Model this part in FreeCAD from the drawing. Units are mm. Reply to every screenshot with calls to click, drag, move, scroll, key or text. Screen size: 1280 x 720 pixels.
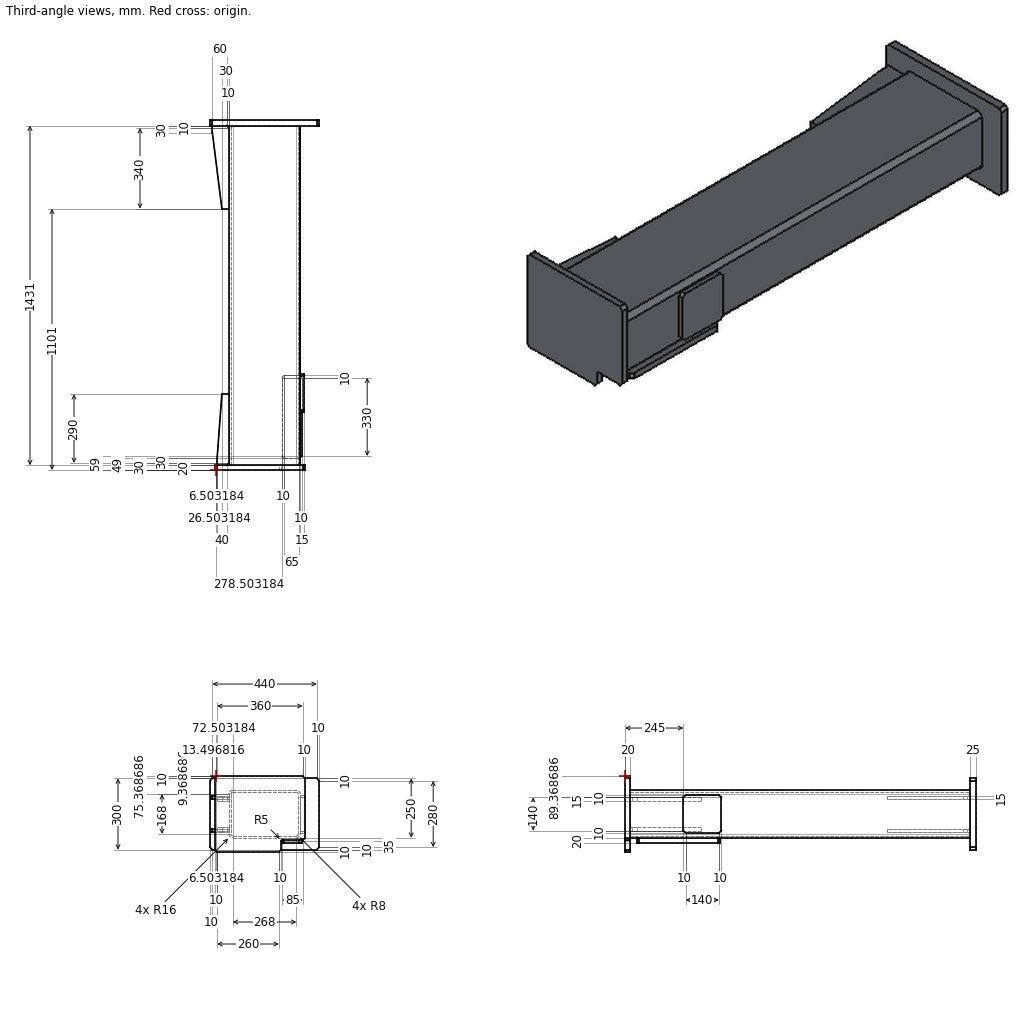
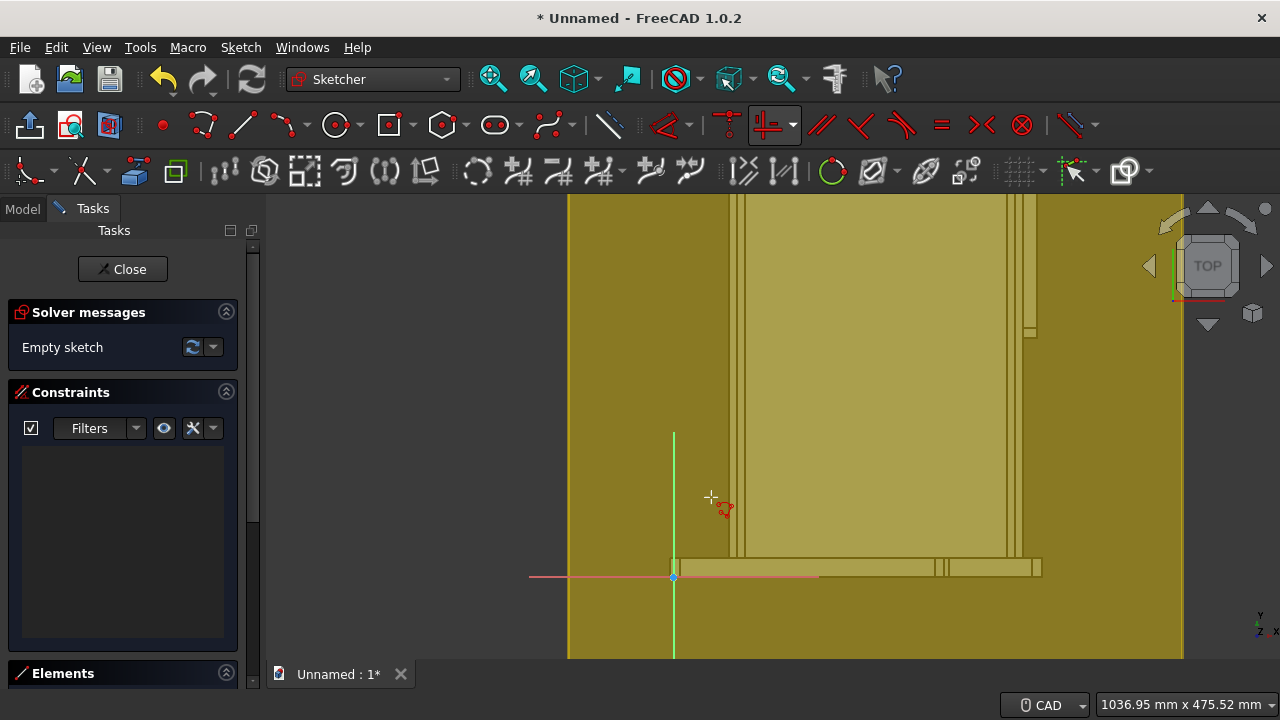
scroll(680, 558, up, 5)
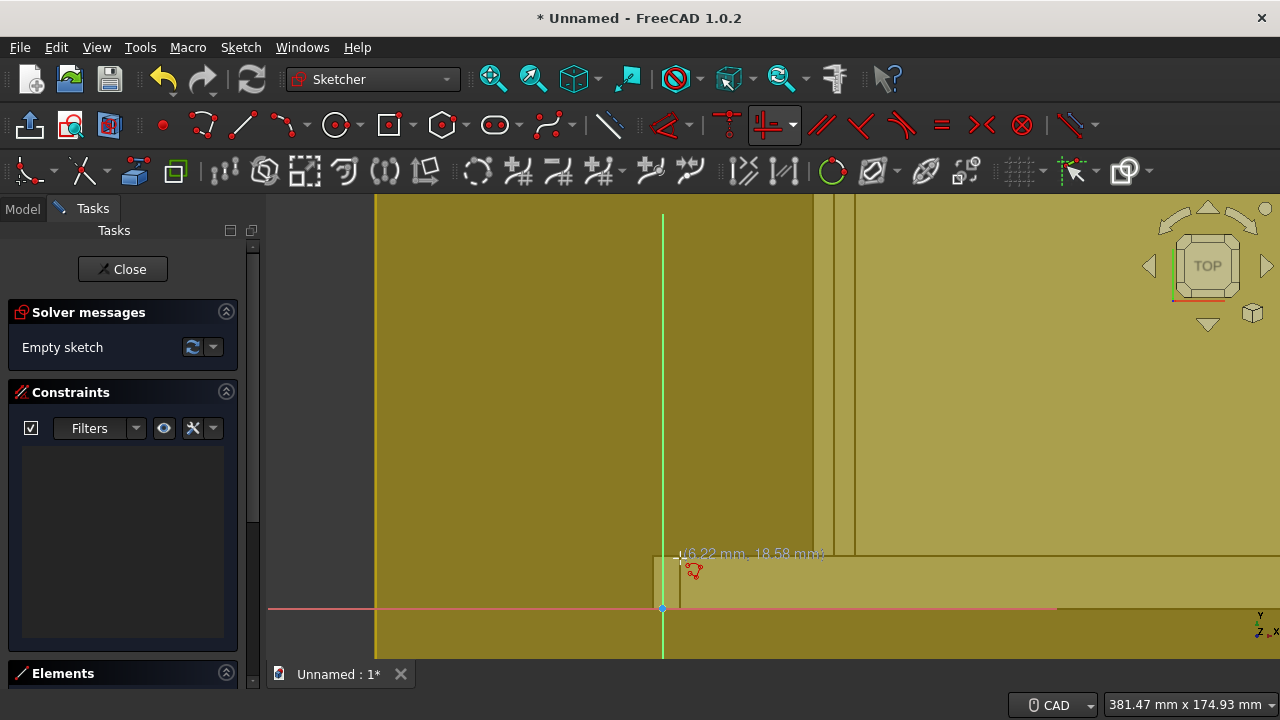
click(680, 556)
click(786, 556)
click(813, 529)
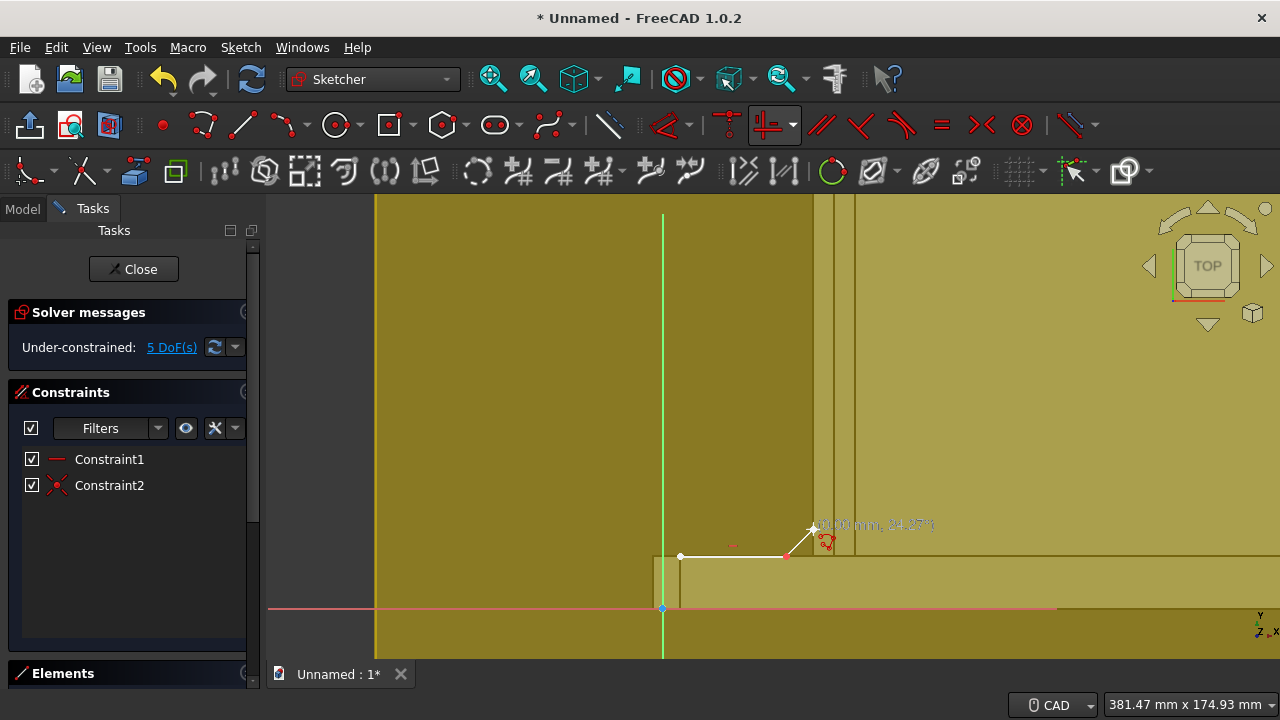
scroll(685, 568, down, 5)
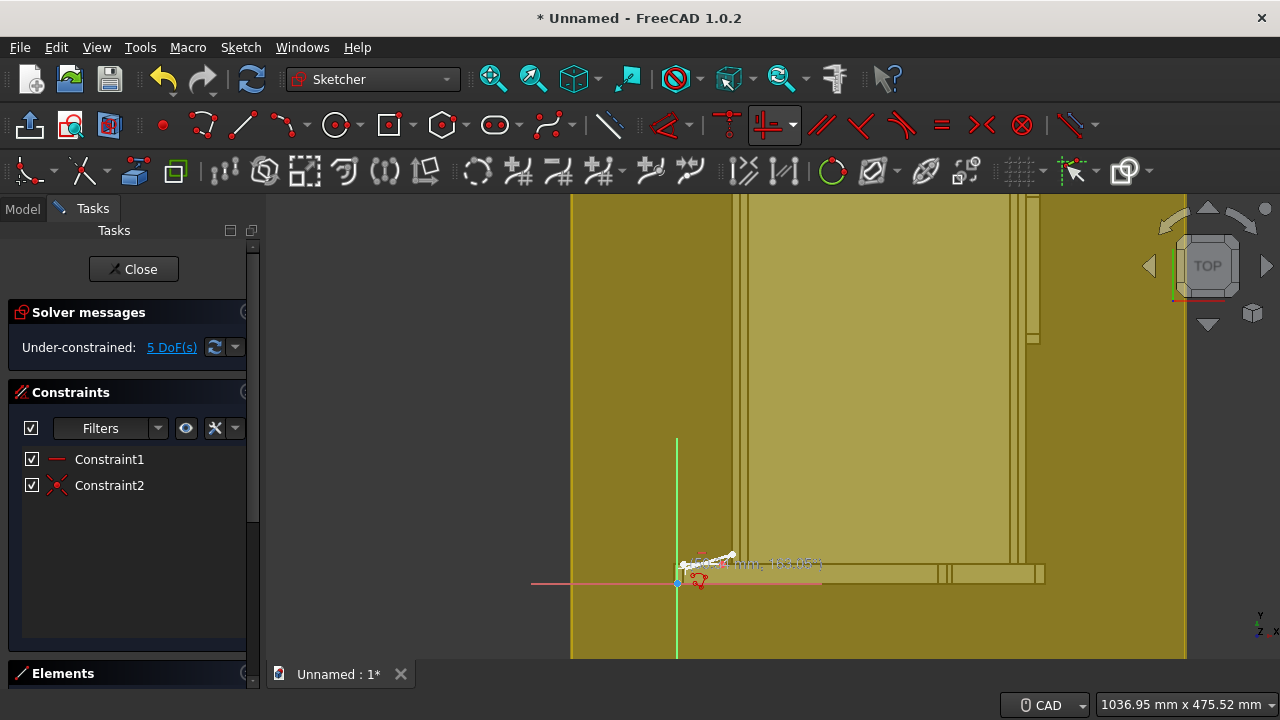
click(732, 271)
click(703, 271)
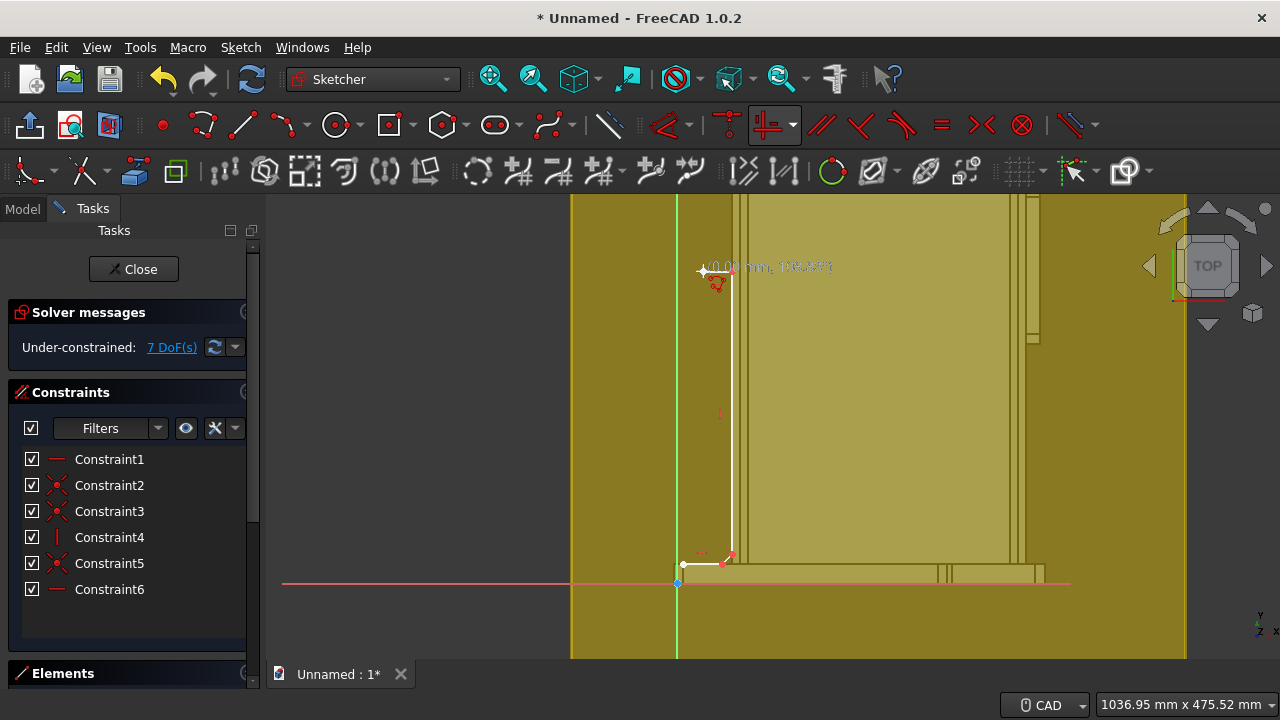
scroll(683, 535, up, 5)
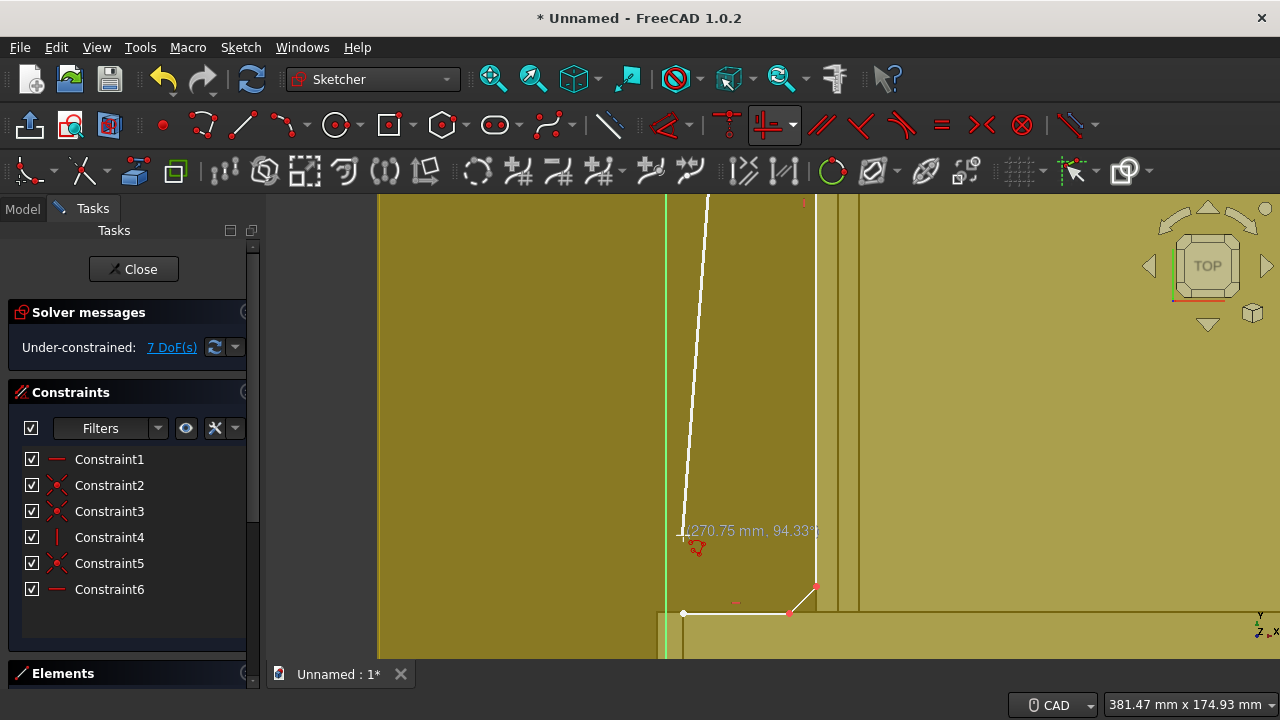
click(683, 533)
click(683, 614)
key(Escape)
key(Escape)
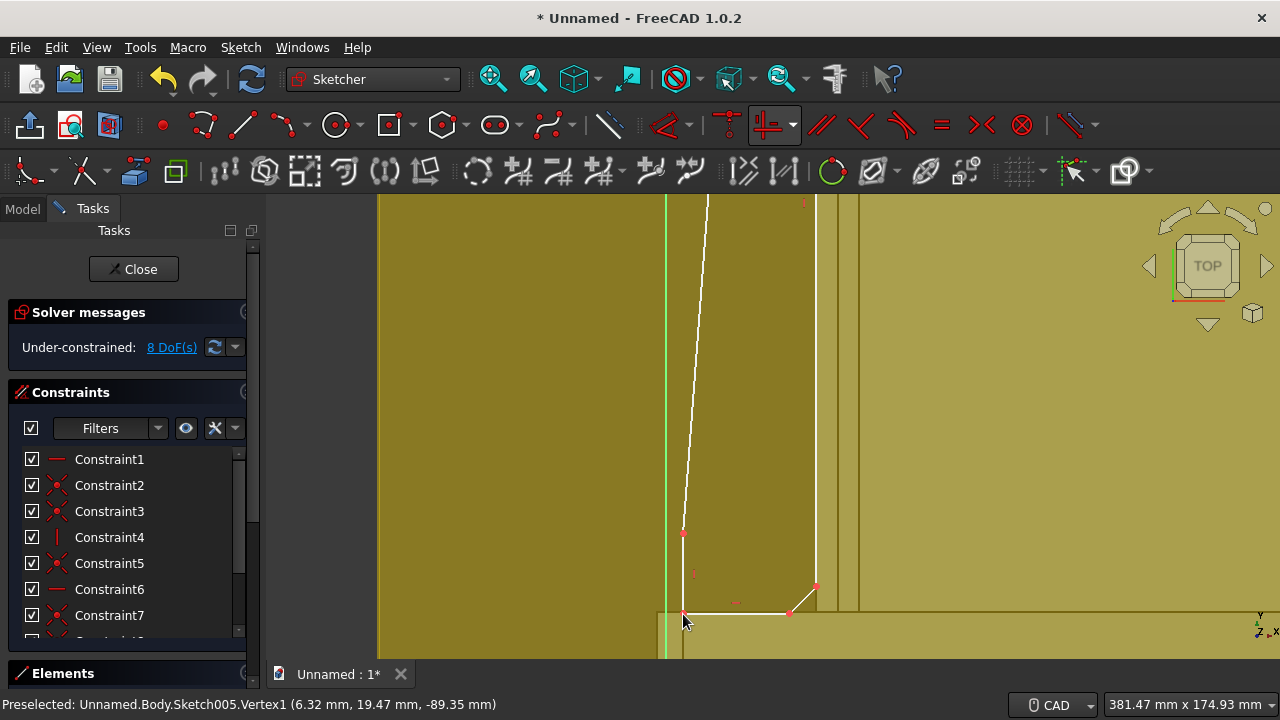
click(664, 126)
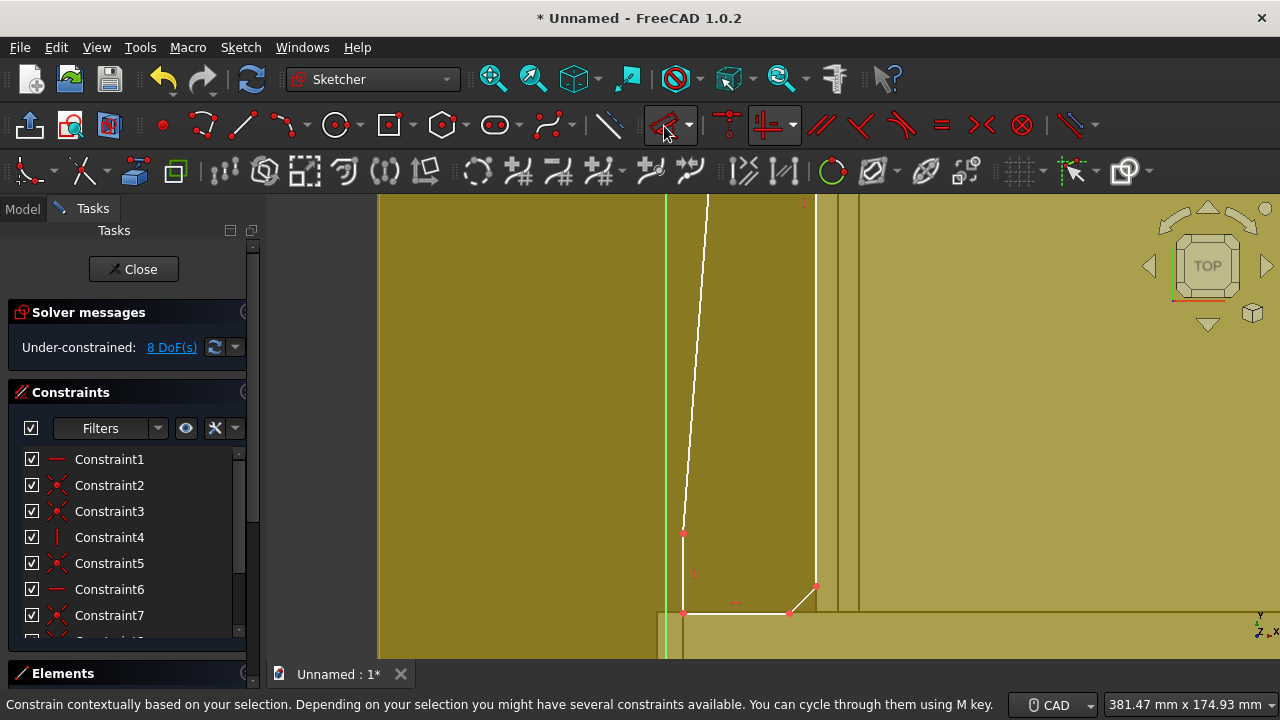
click(715, 614)
click(736, 580)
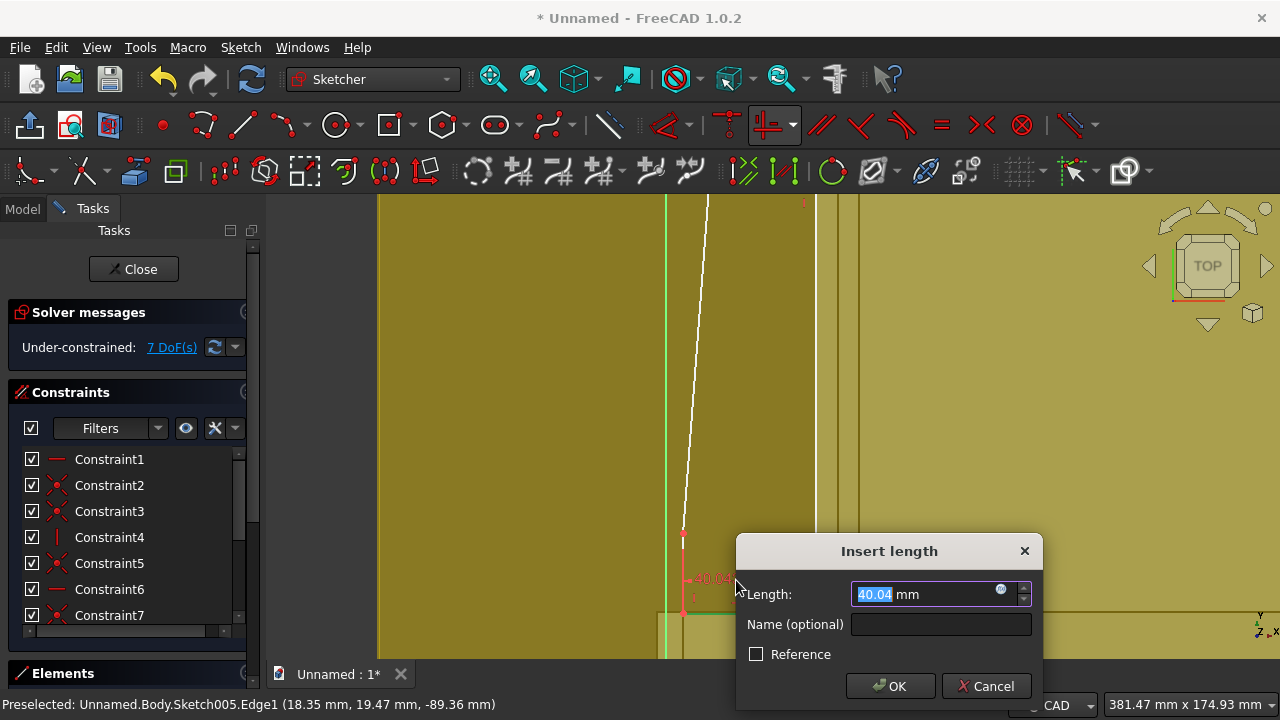
text(40)
key(Return)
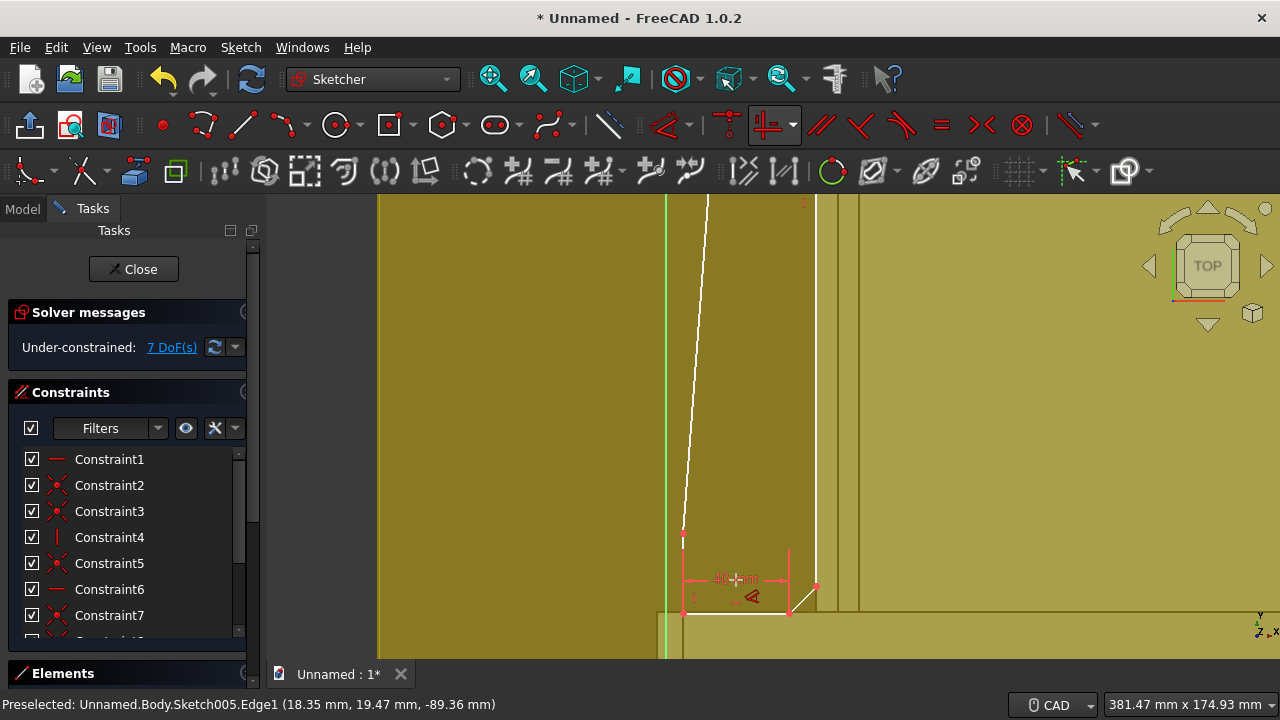
scroll(683, 535, down, 5)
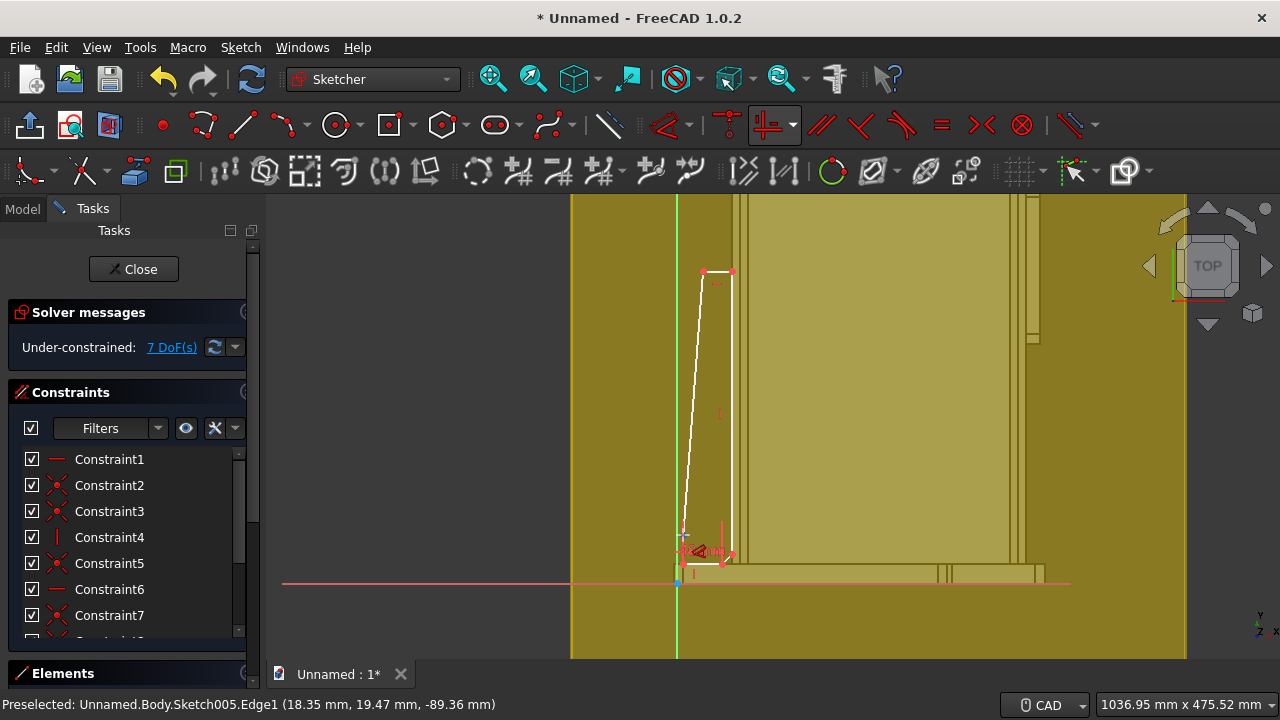
scroll(724, 272, up, 3)